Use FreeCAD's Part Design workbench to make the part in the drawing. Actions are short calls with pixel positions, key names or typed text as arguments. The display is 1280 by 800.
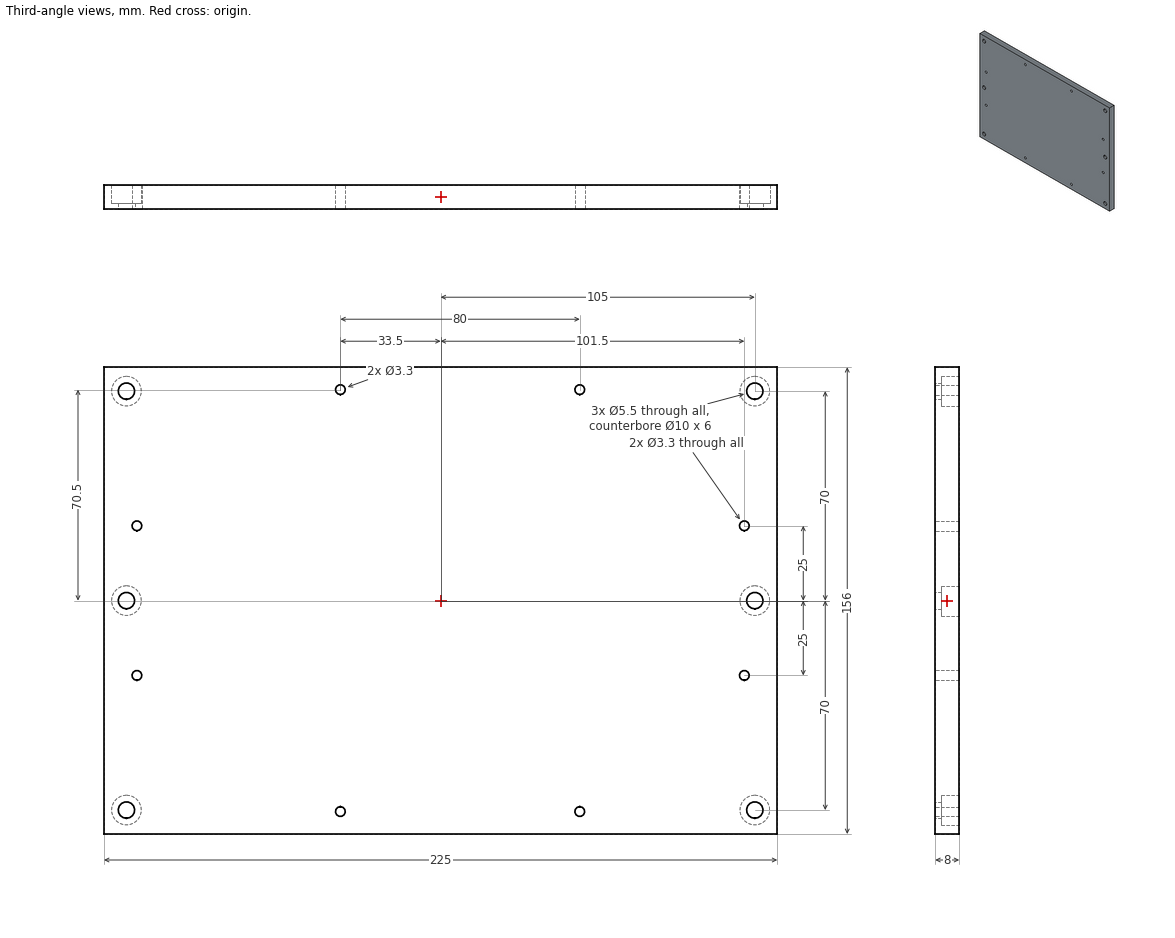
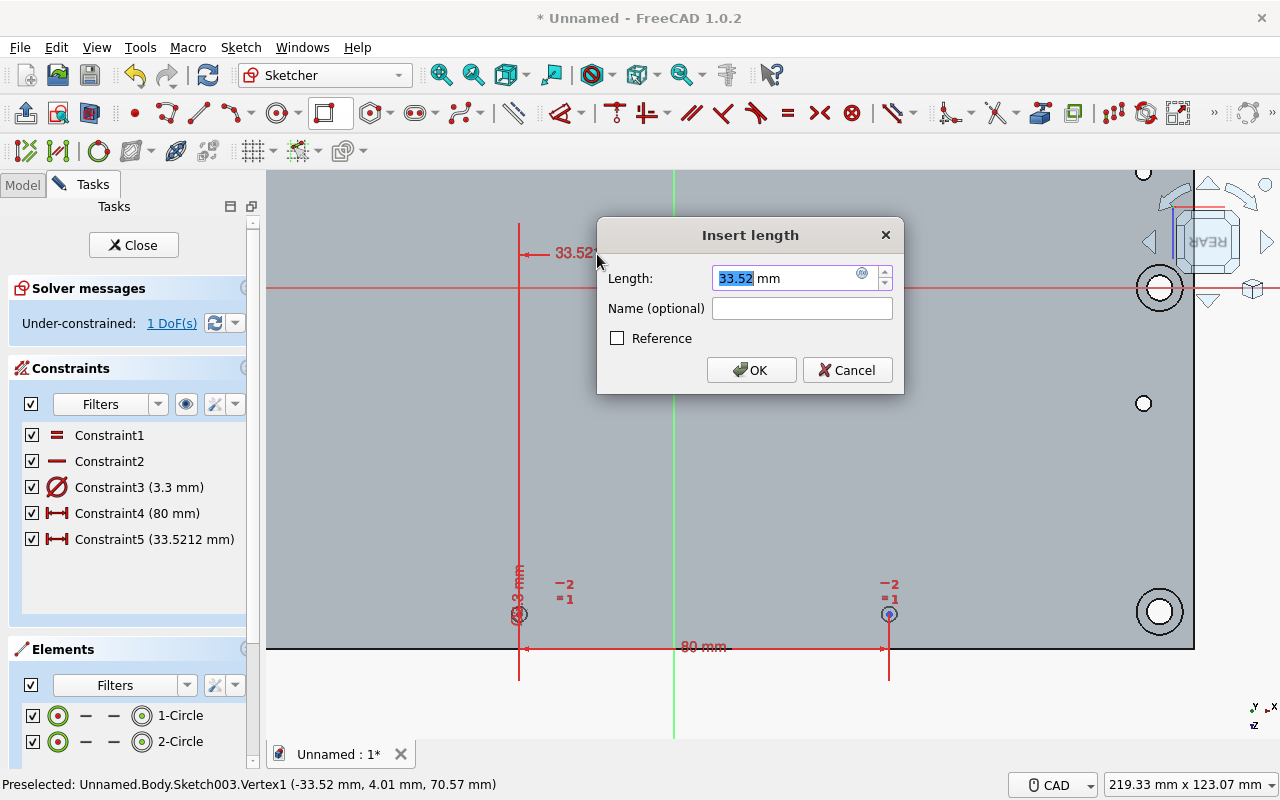
text(33.5)
key(Return)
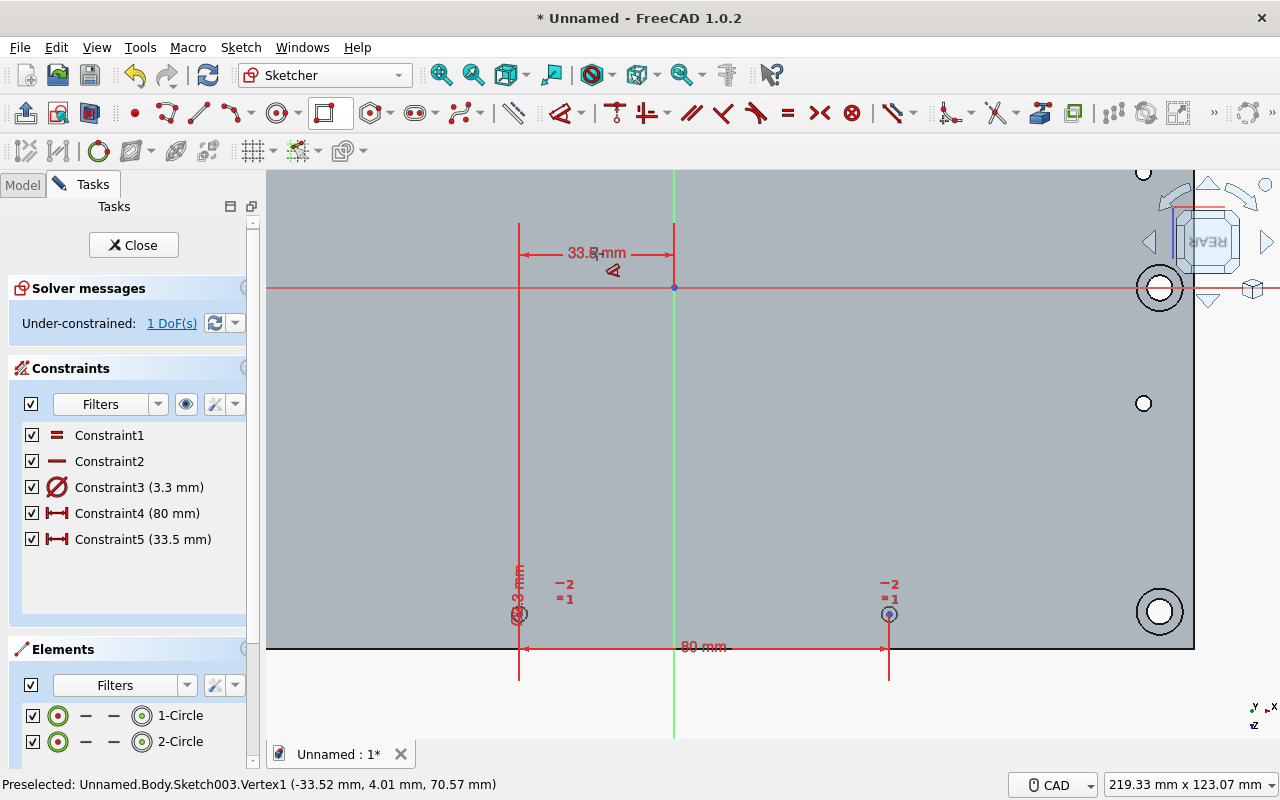
click(519, 614)
click(485, 451)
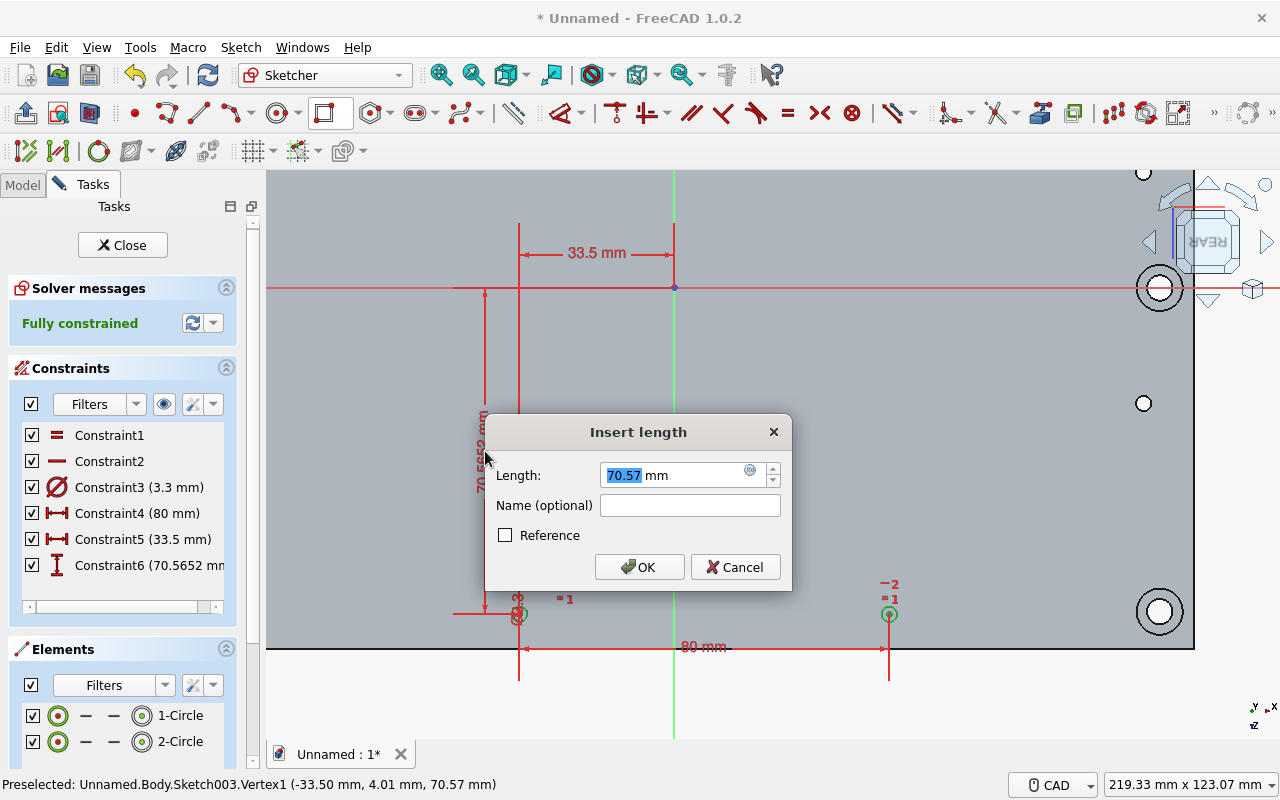
text(70.5)
key(Return)
key(Escape)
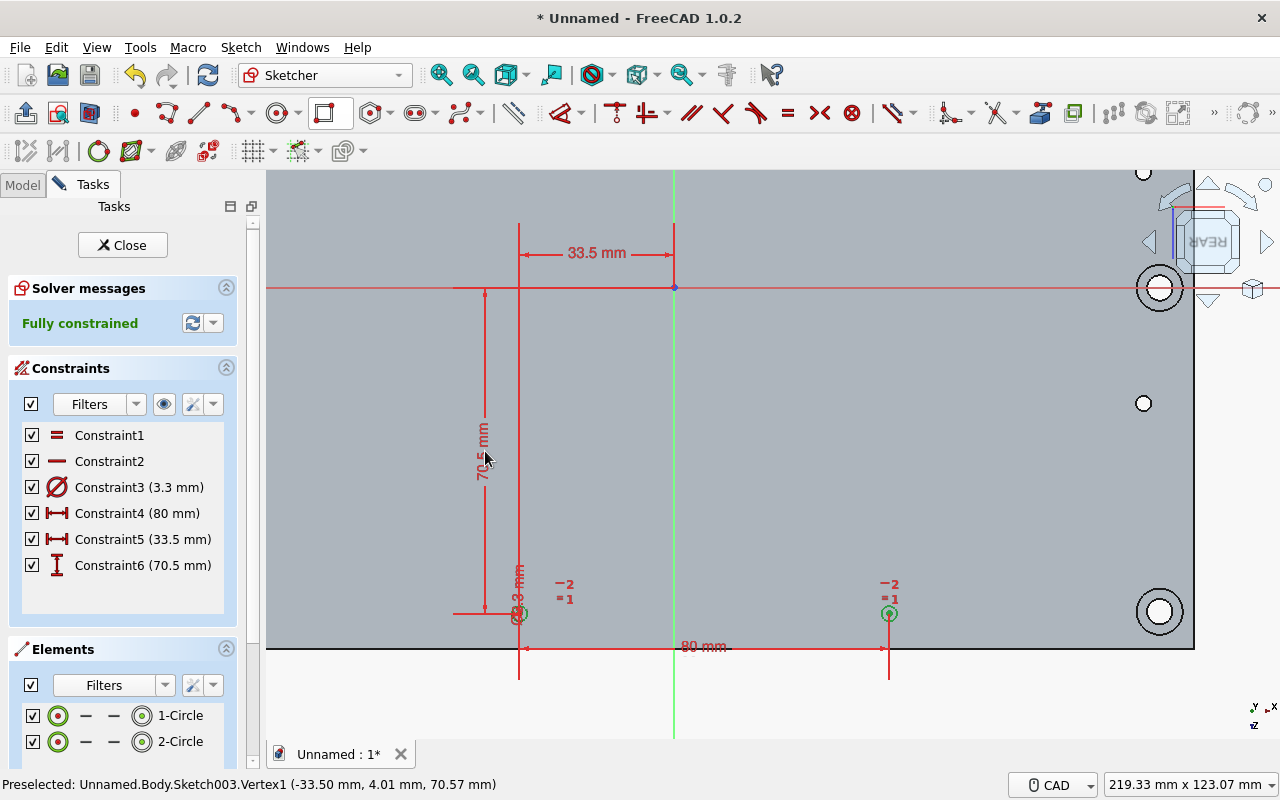
click(123, 245)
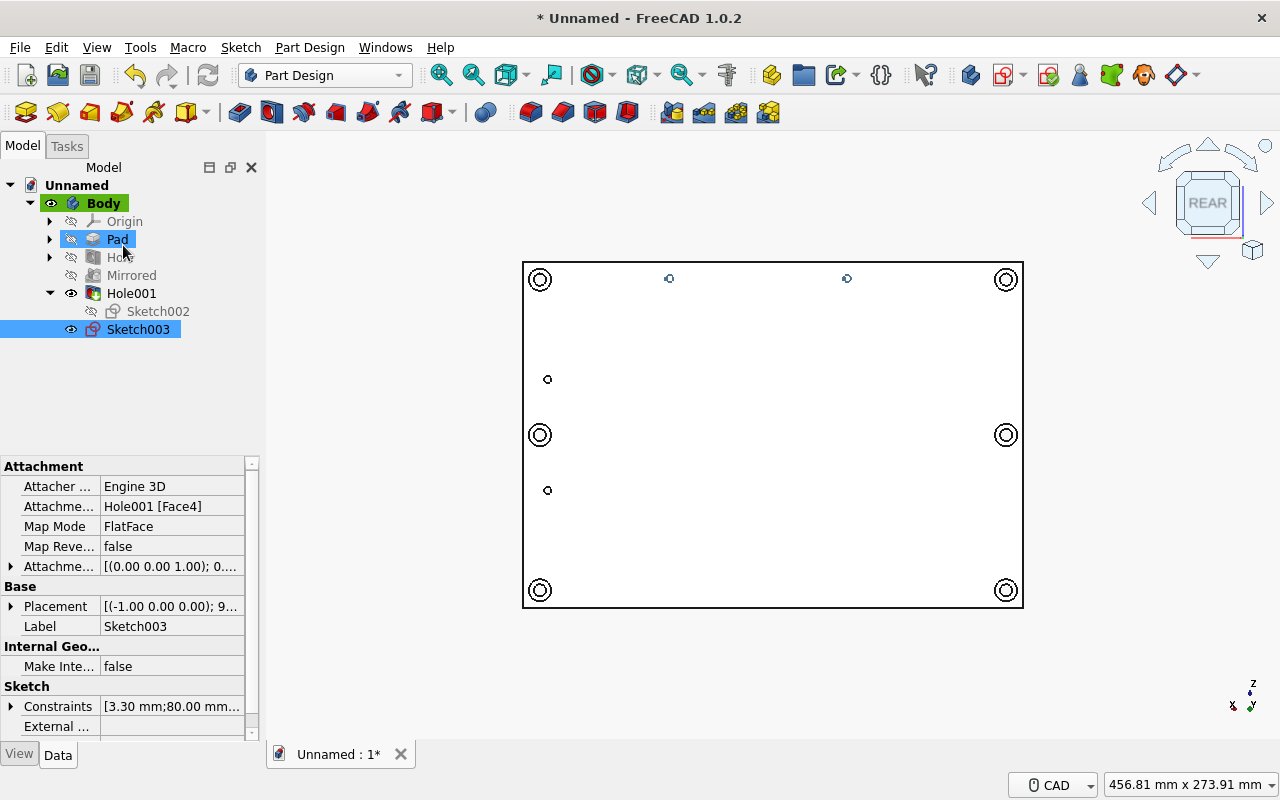
click(240, 112)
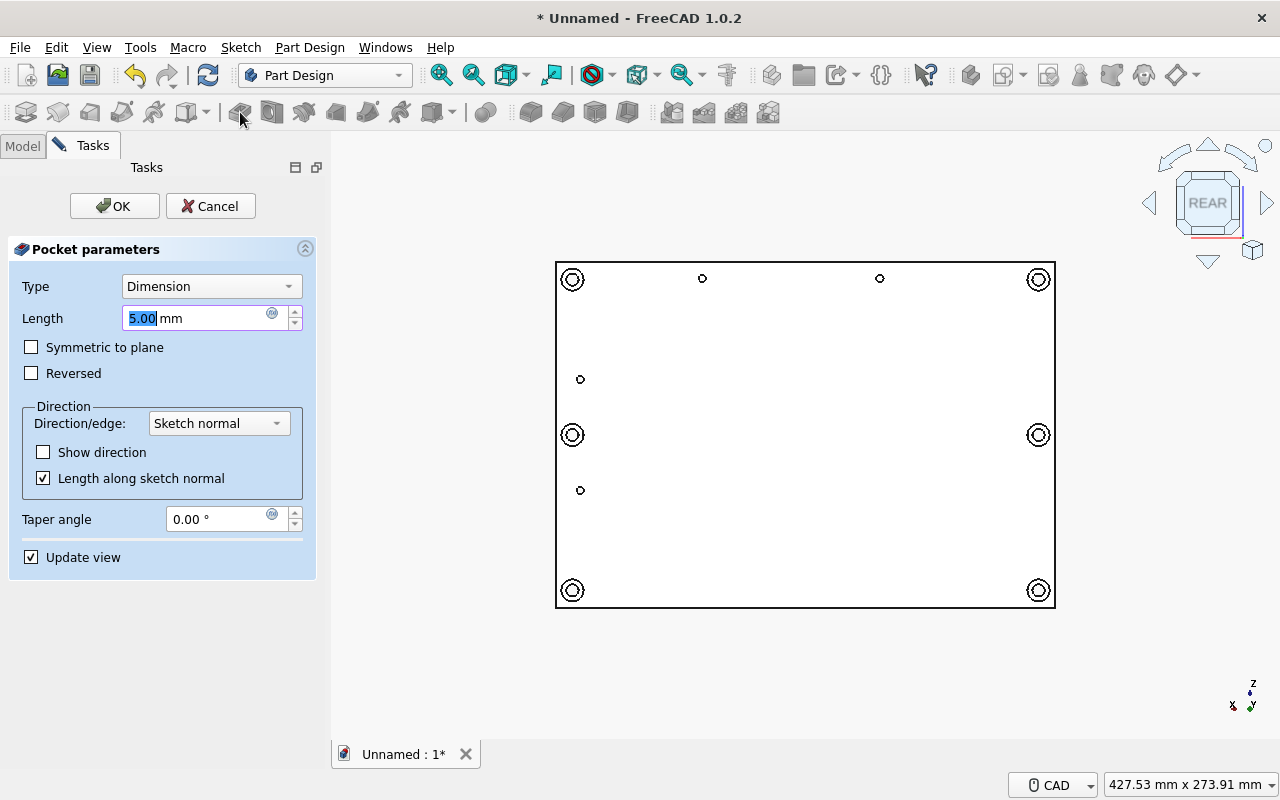
click(212, 286)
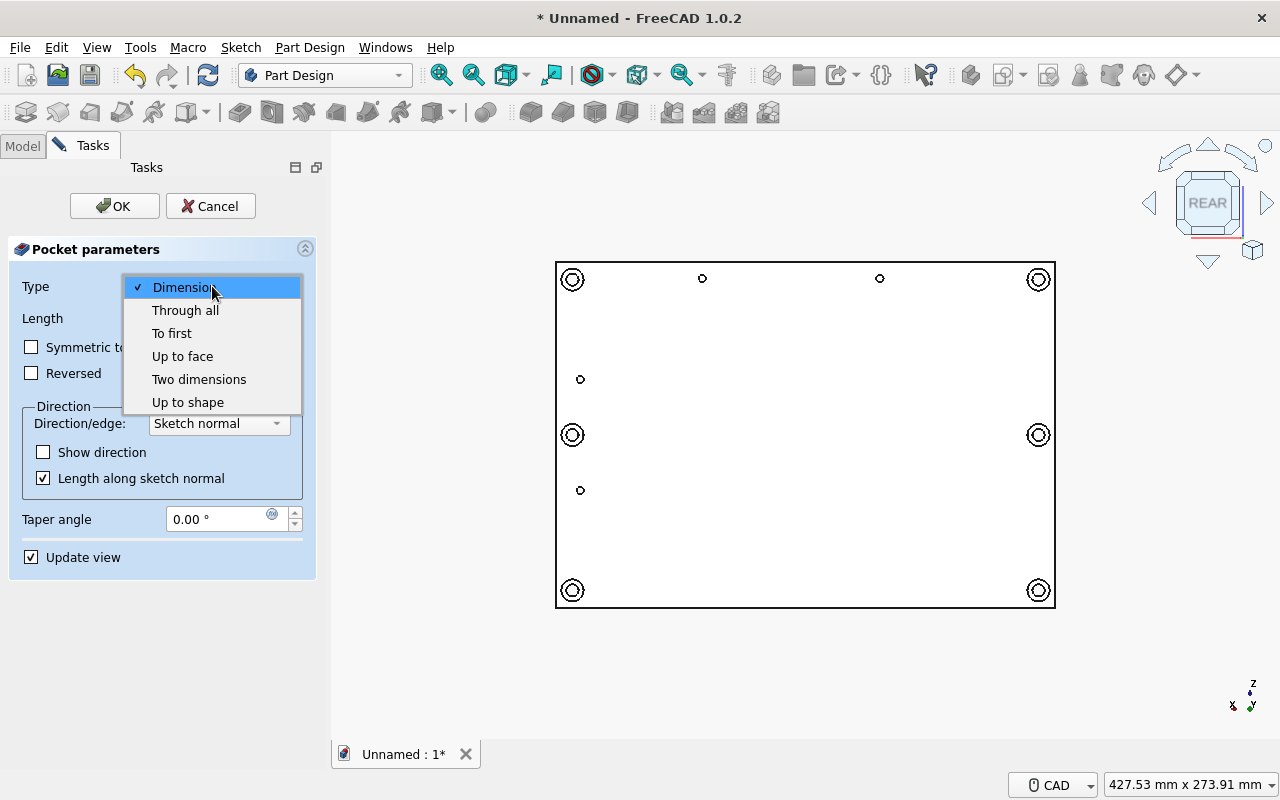
click(212, 310)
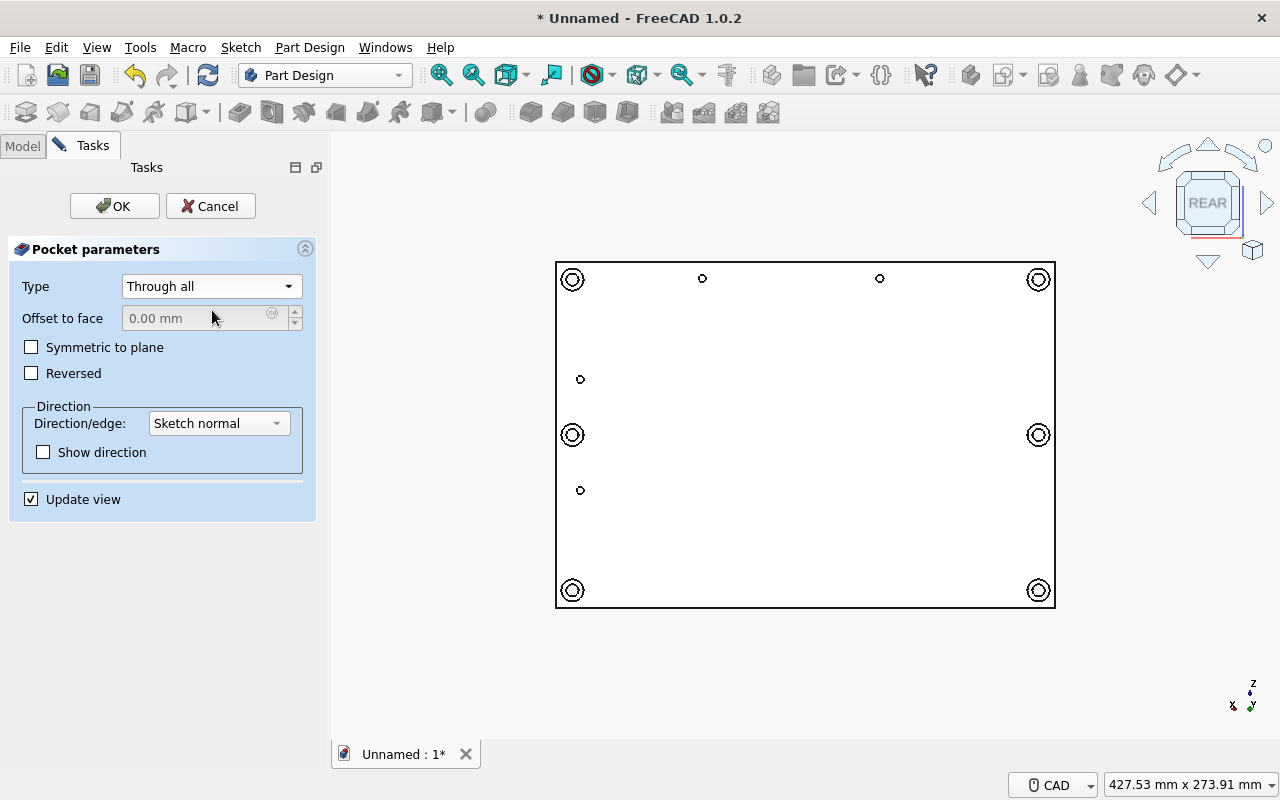
click(115, 206)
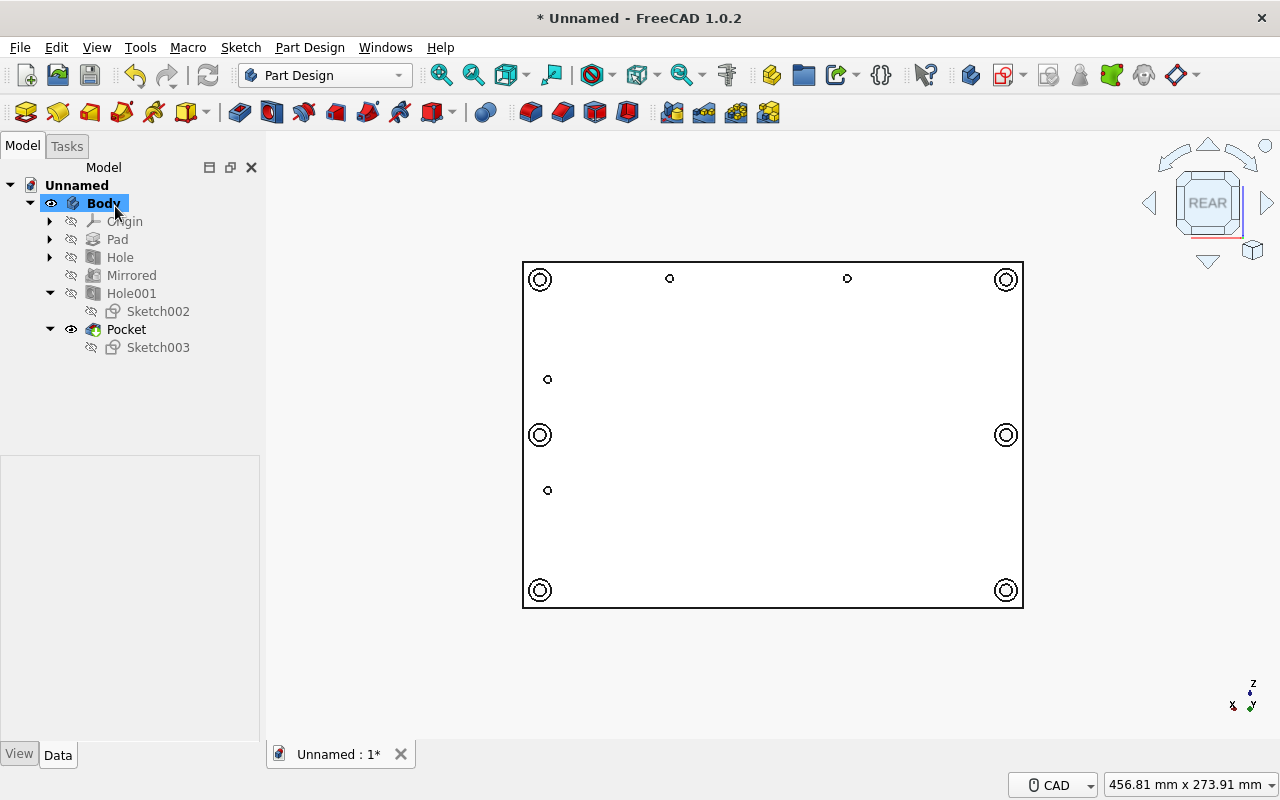
click(116, 293)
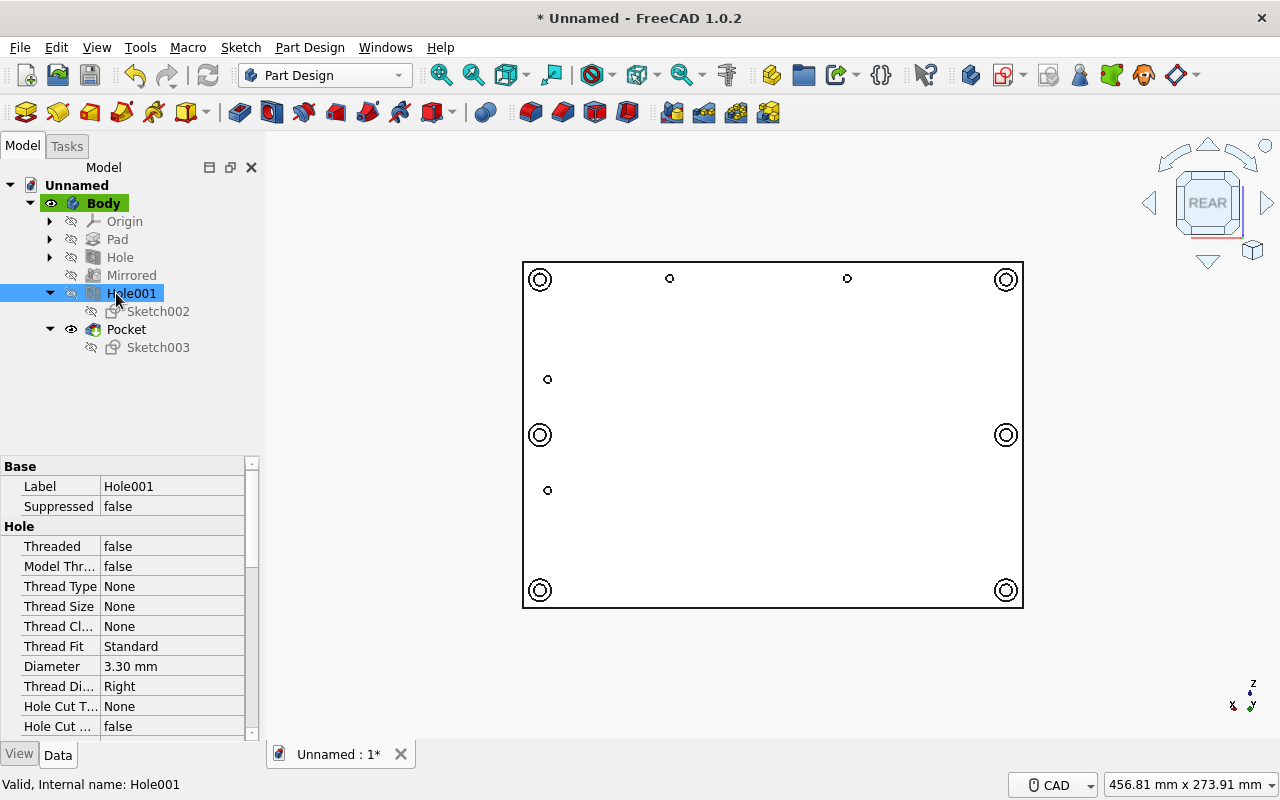
click(672, 112)